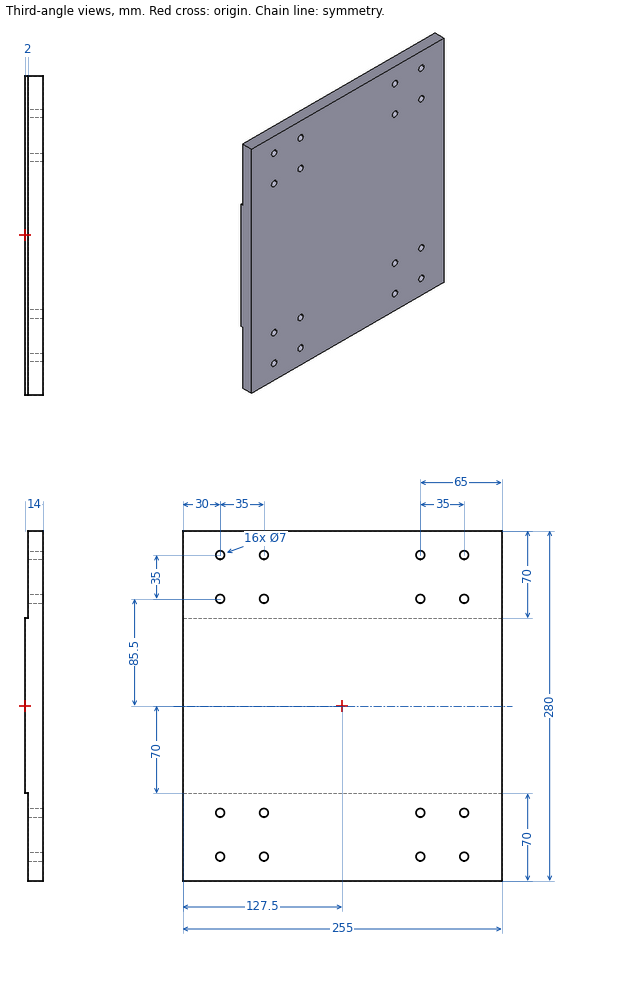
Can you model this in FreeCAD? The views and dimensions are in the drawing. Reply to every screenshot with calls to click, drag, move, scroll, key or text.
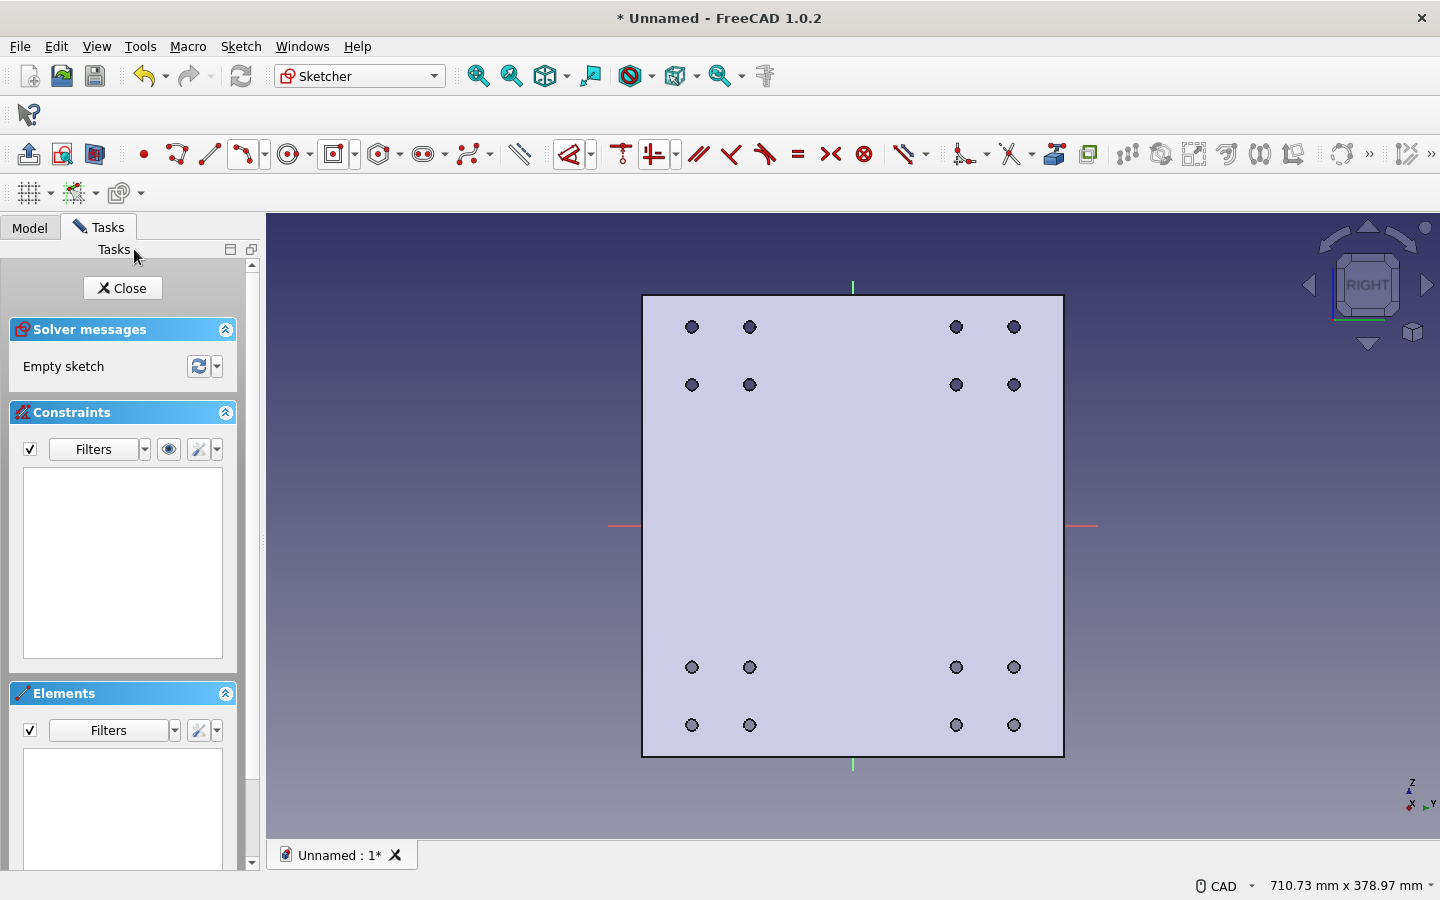
click(95, 154)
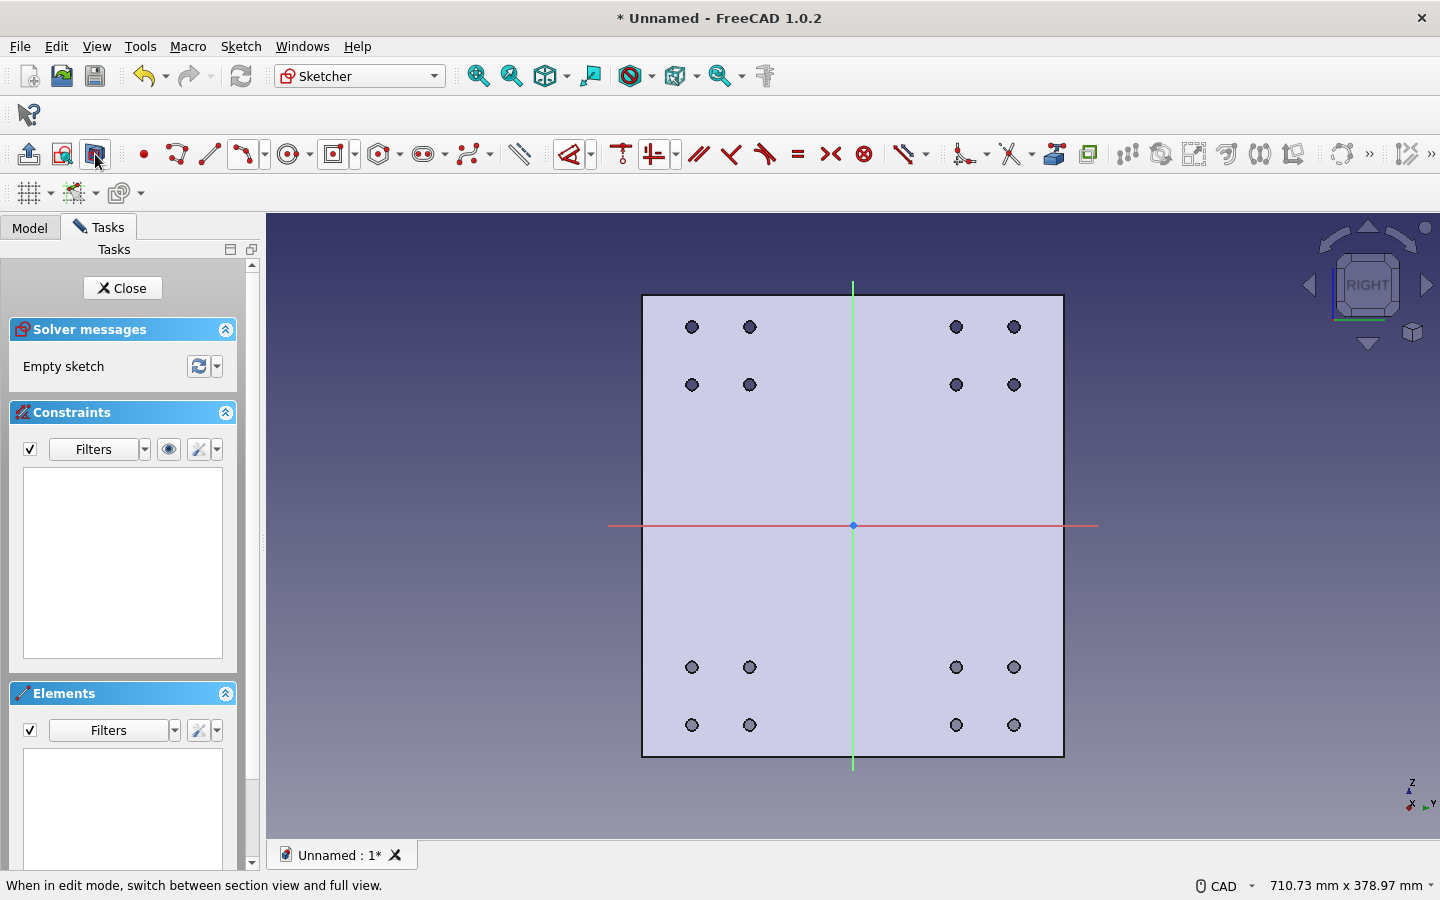
key(g)
key(r)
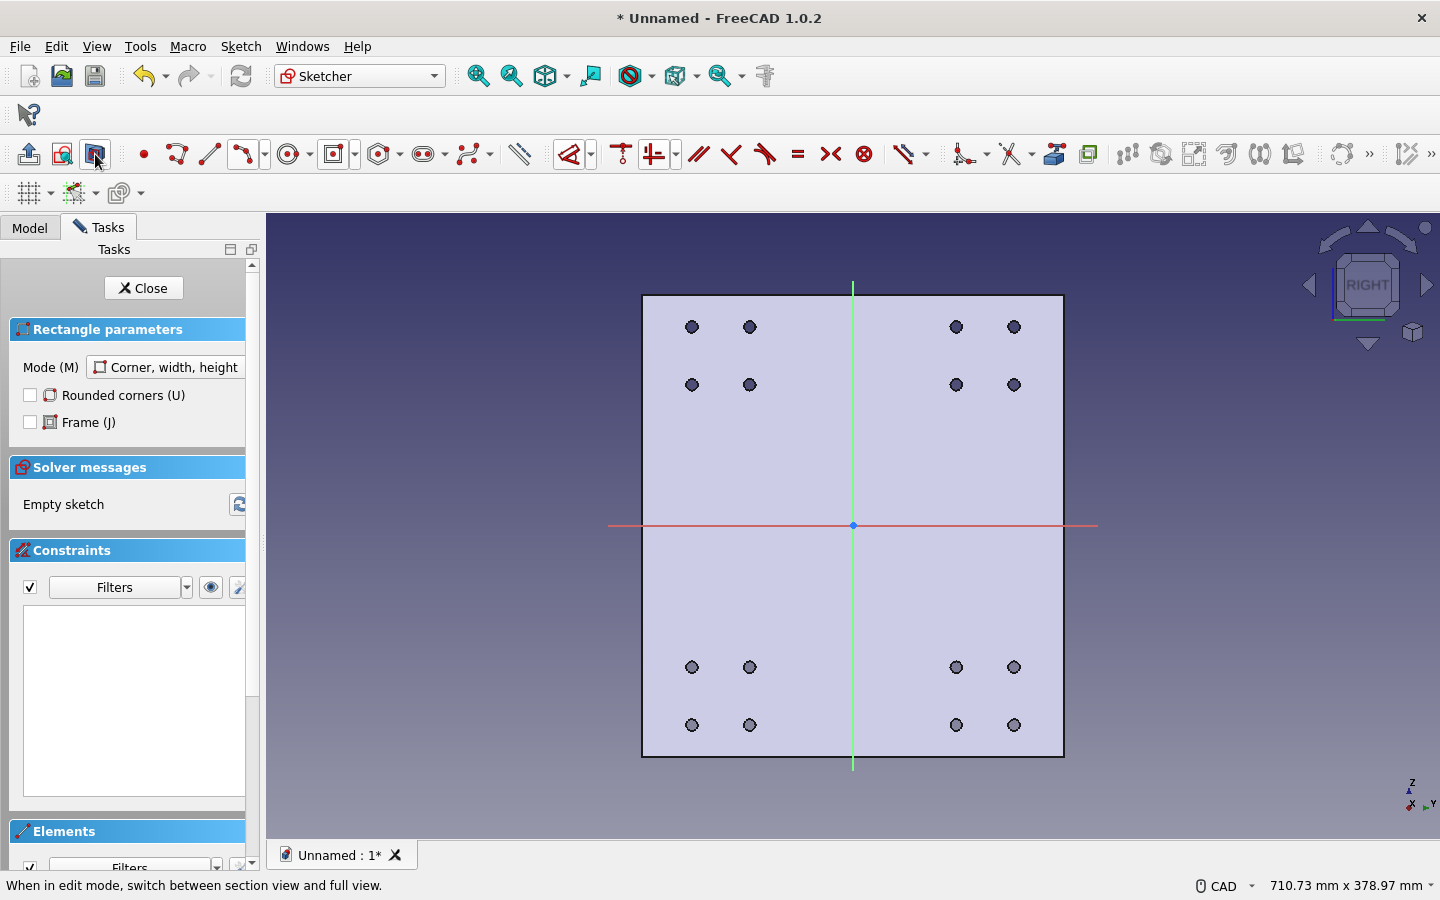
click(642, 642)
move(1064, 757)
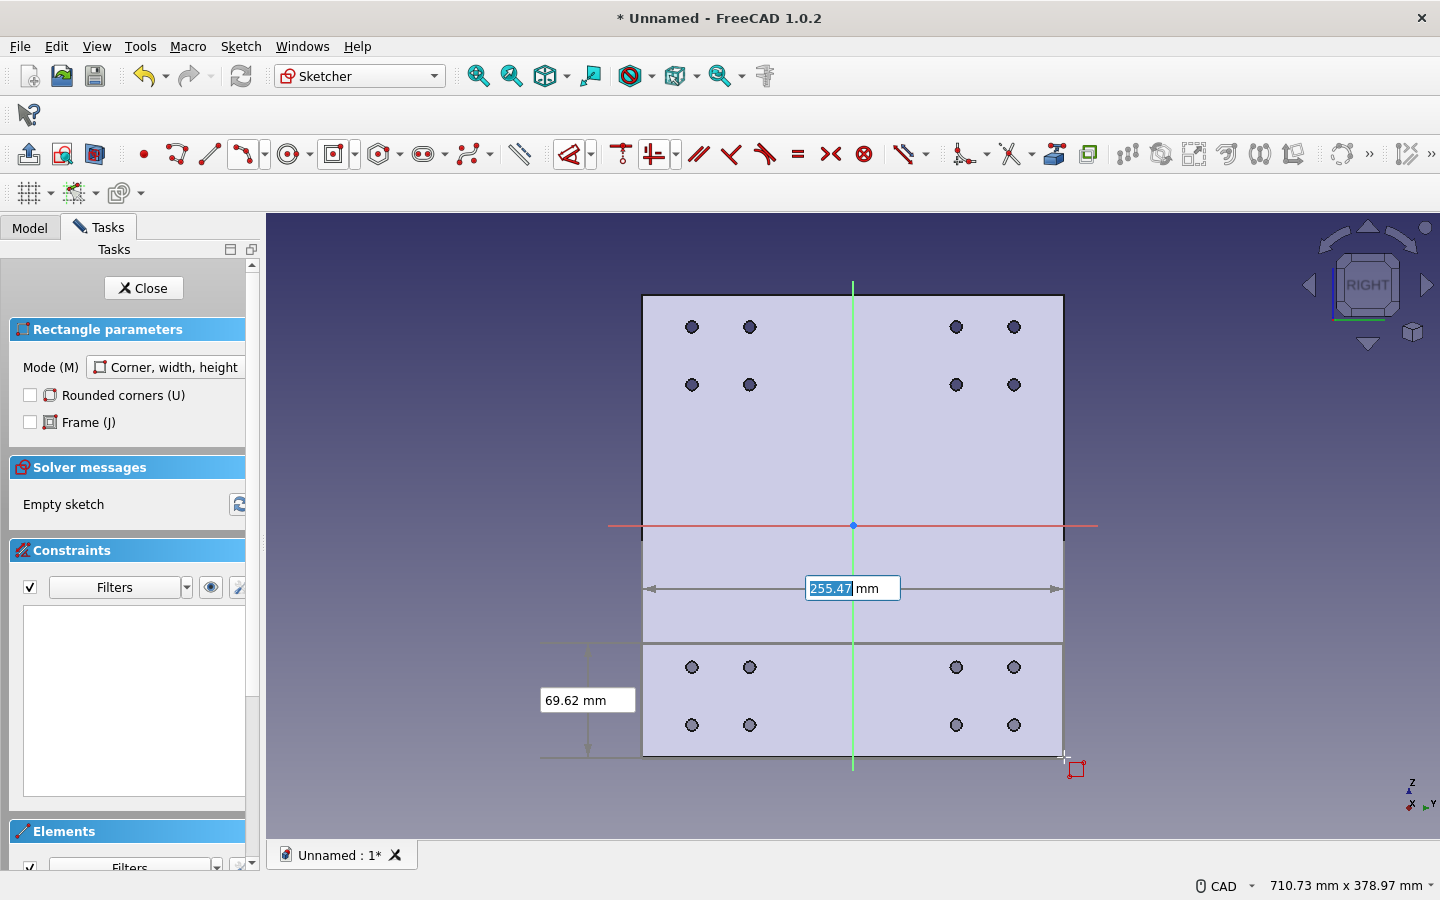
text(255)
key(Tab)
text(70)
key(Return)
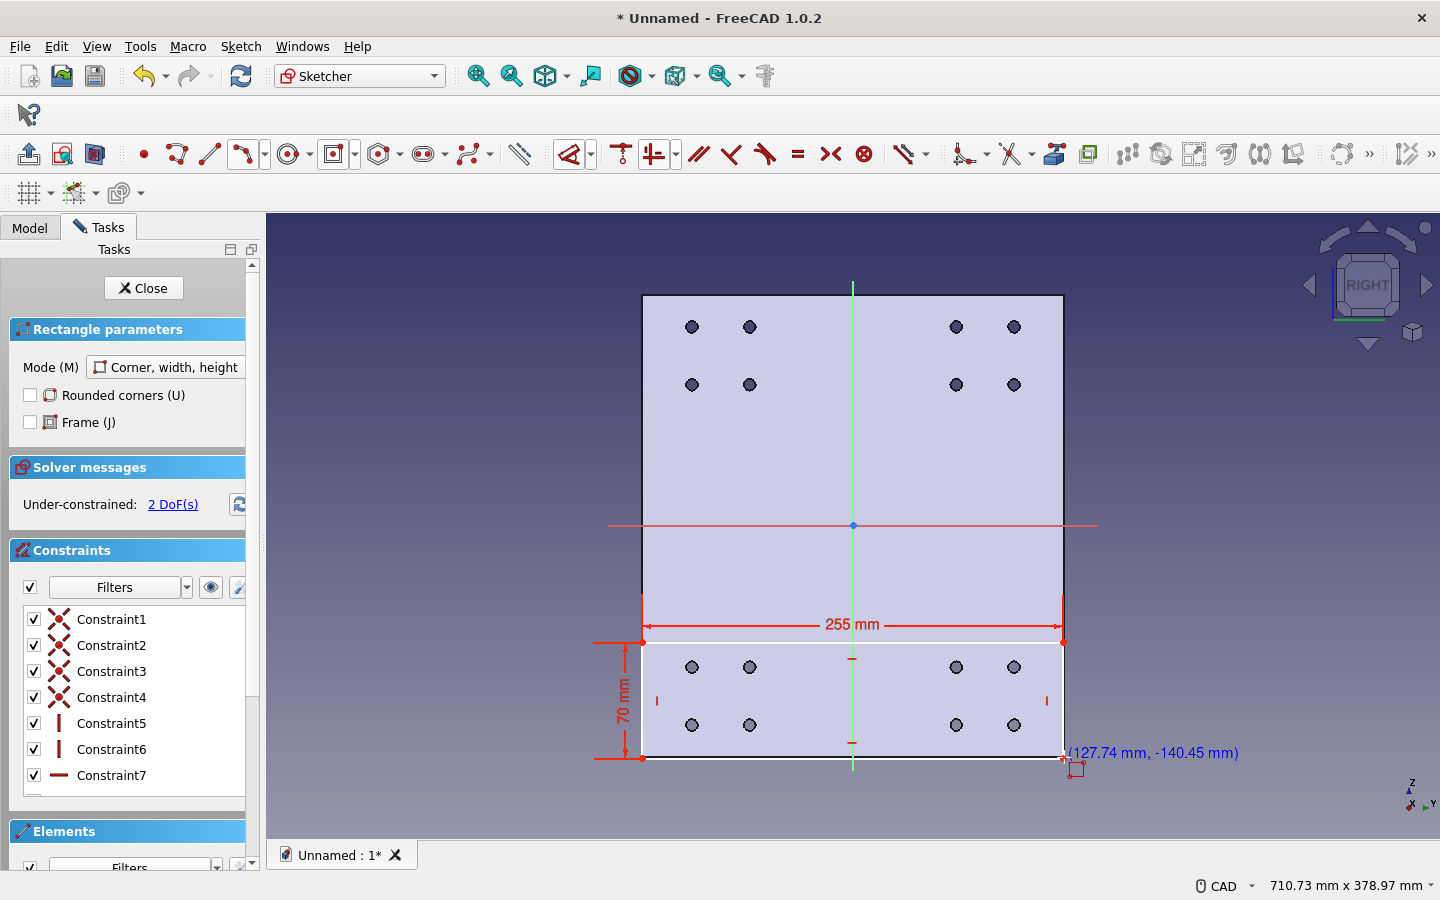
click(642, 295)
move(1064, 410)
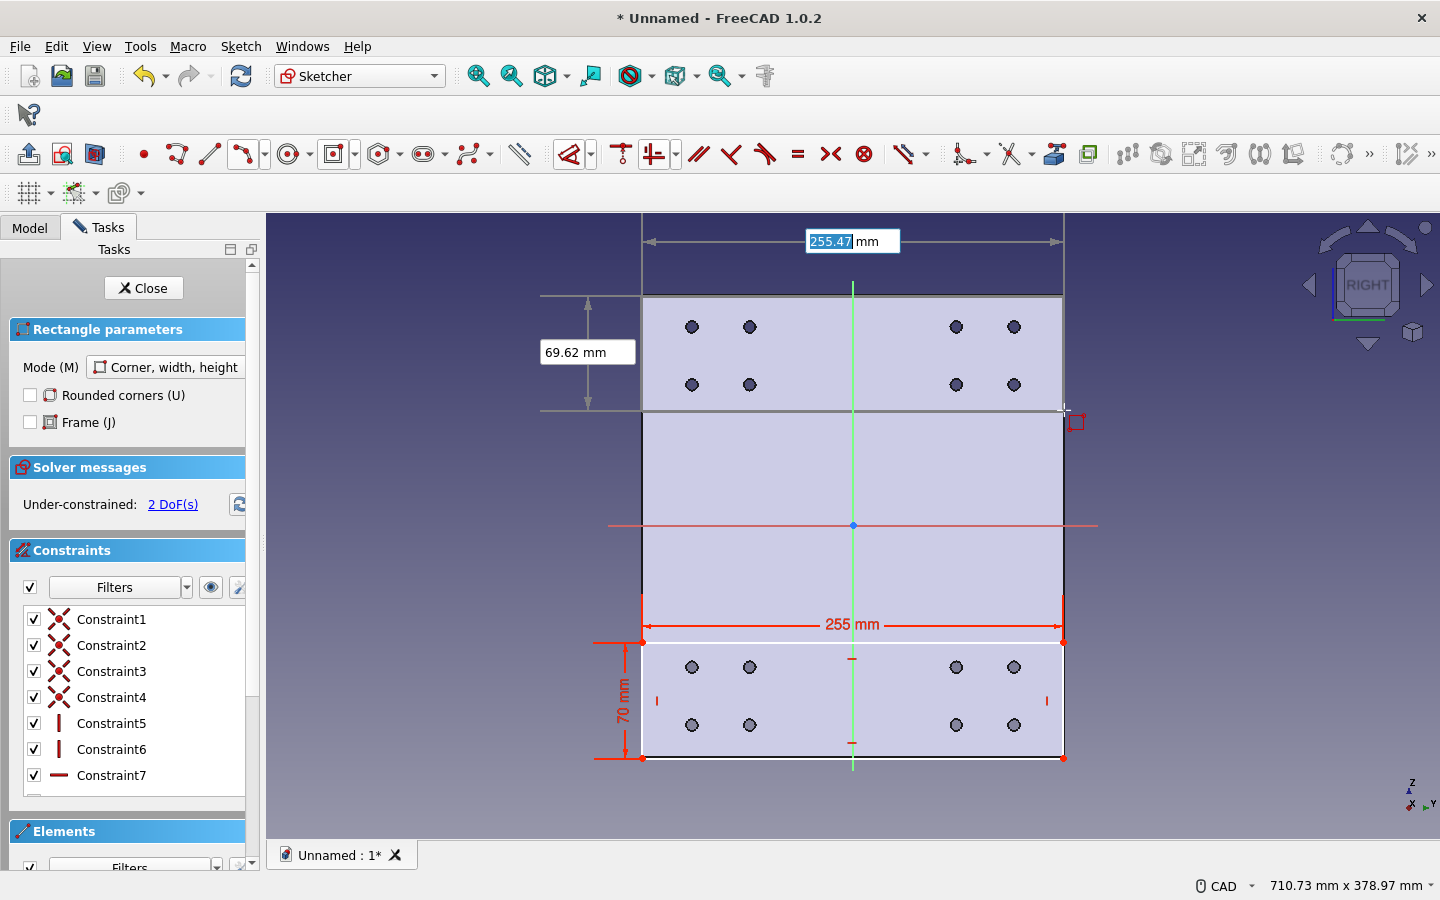
text(255)
key(Tab)
text(70)
key(Return)
key(Escape)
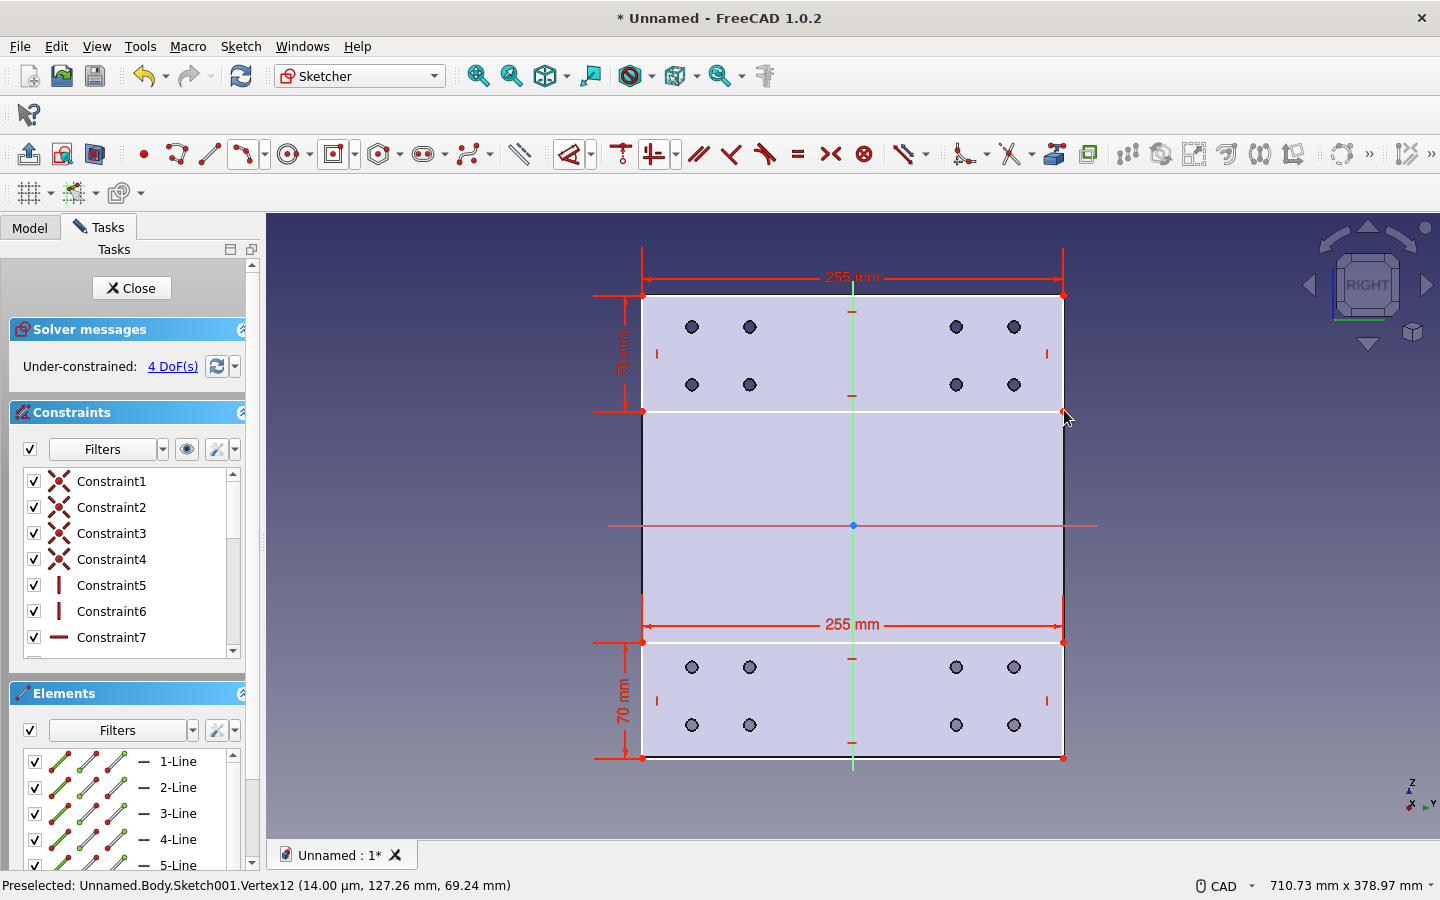
click(642, 759)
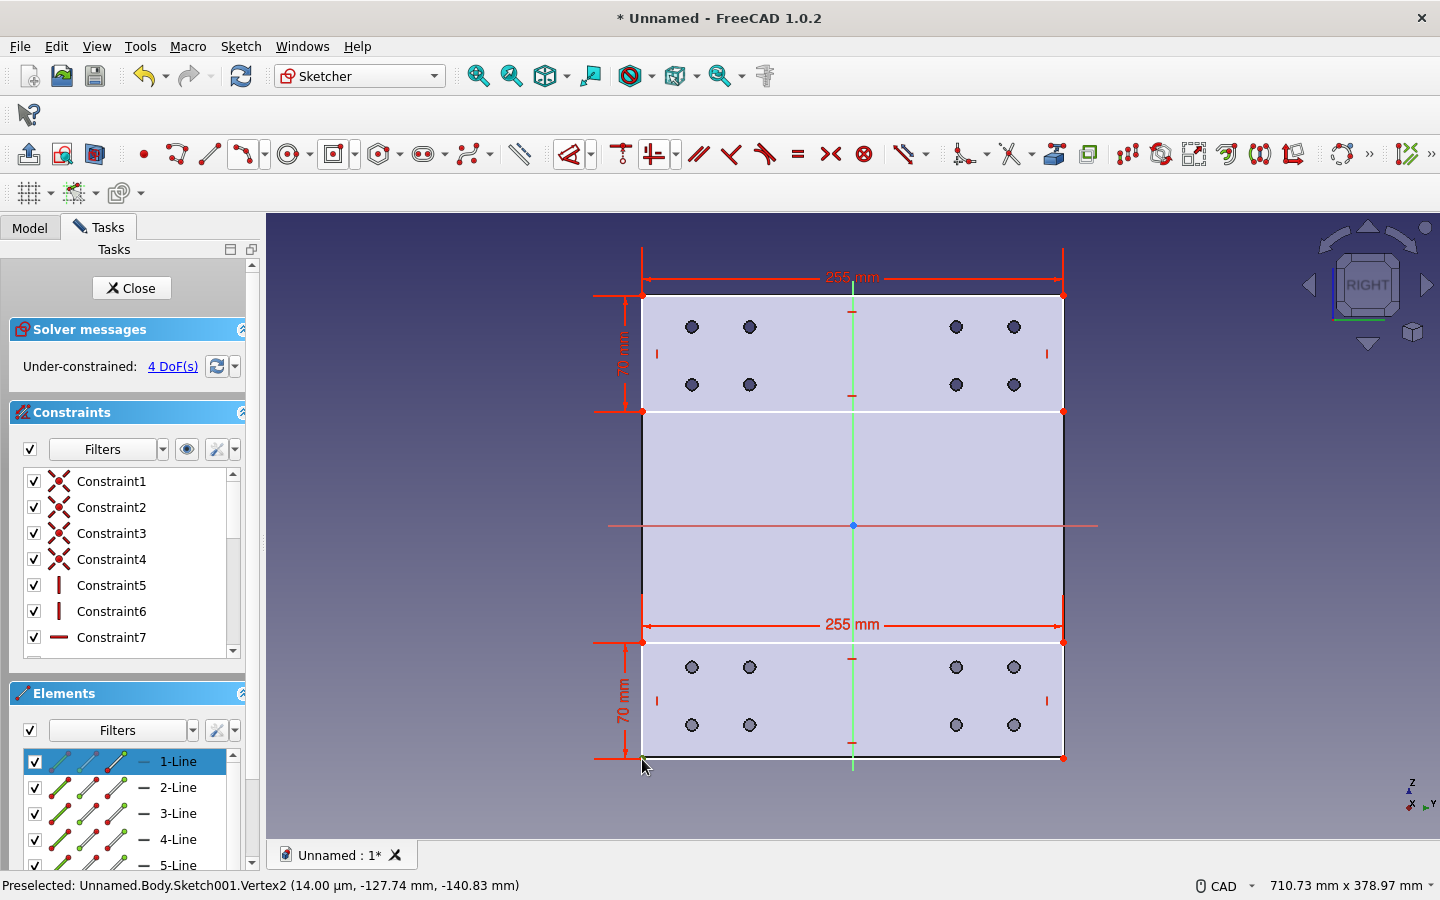
click(642, 296)